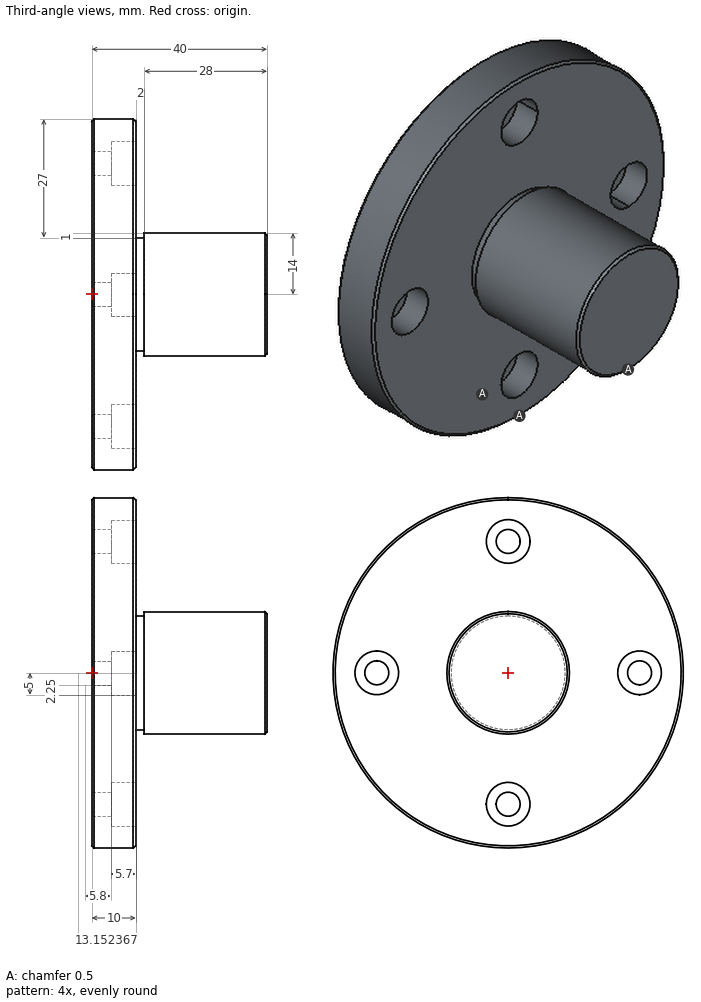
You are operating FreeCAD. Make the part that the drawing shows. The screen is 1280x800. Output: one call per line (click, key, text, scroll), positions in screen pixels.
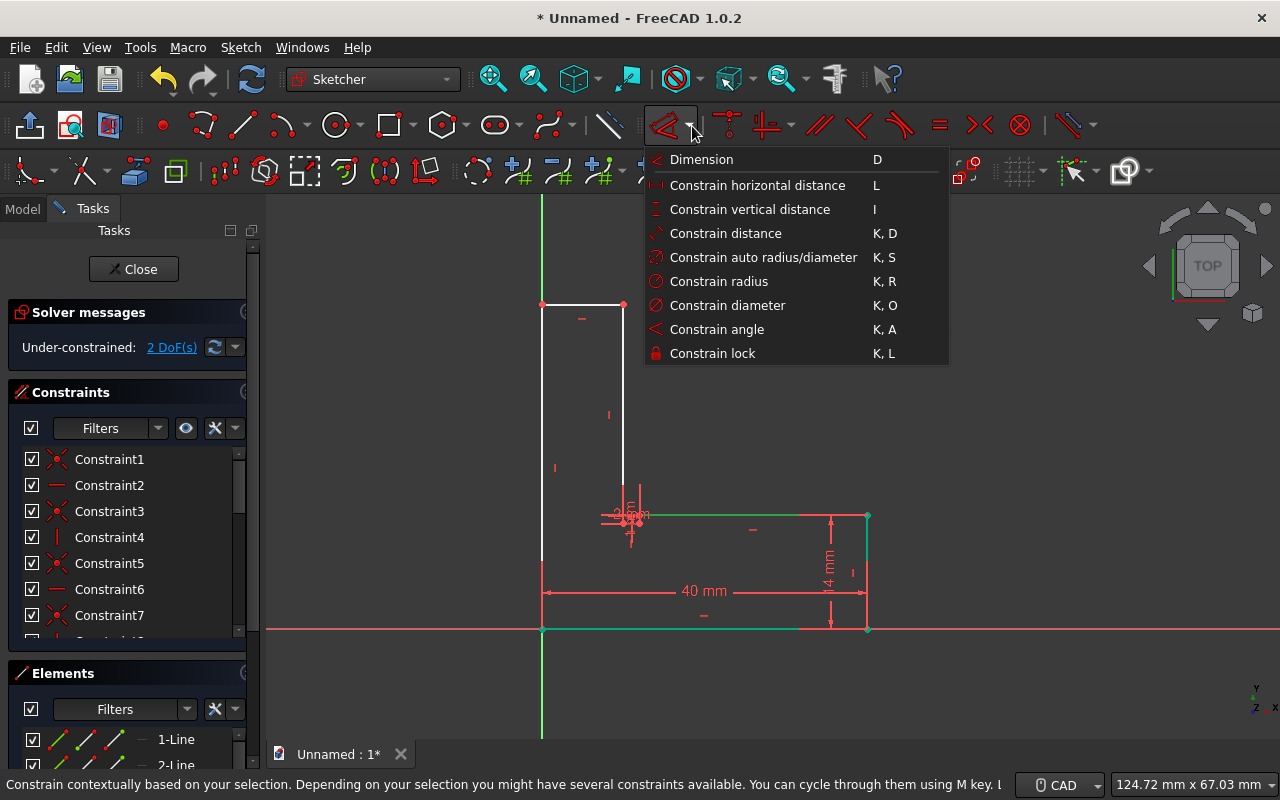
click(797, 185)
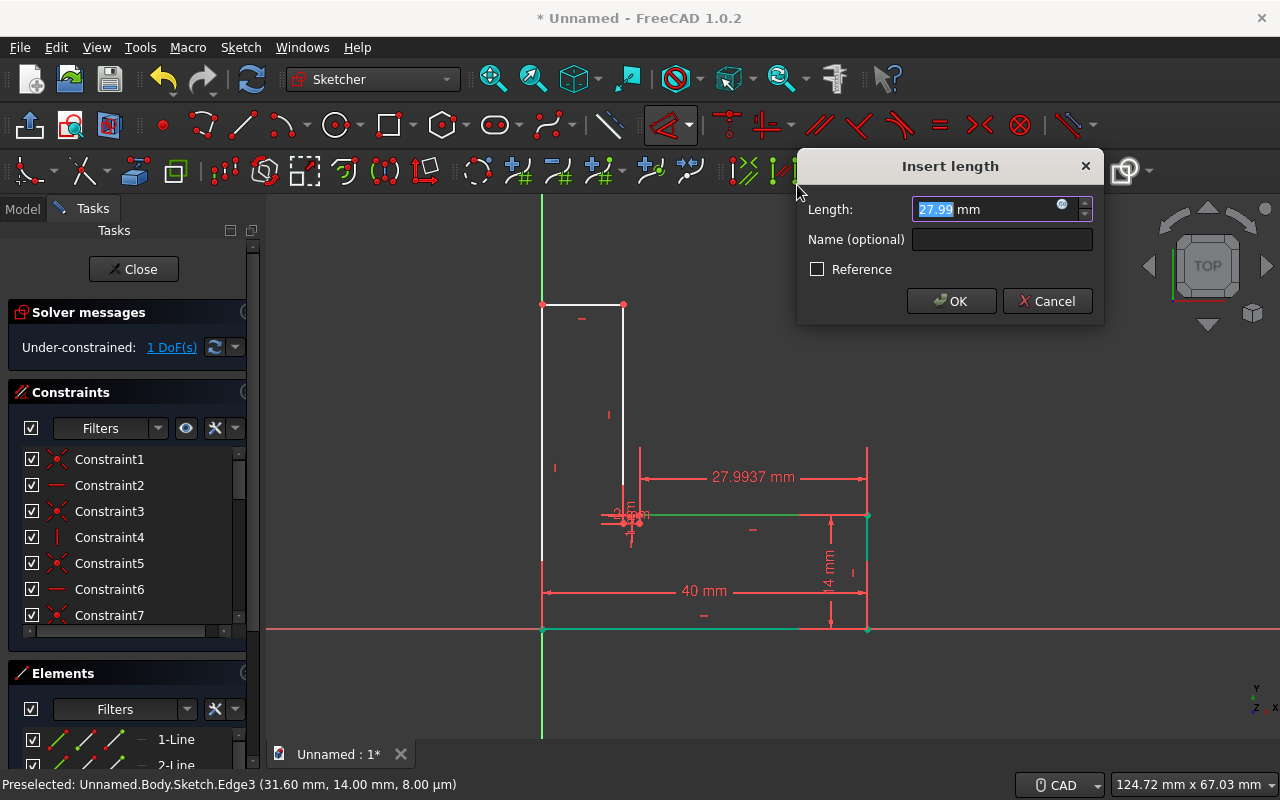
text(28)
key(Return)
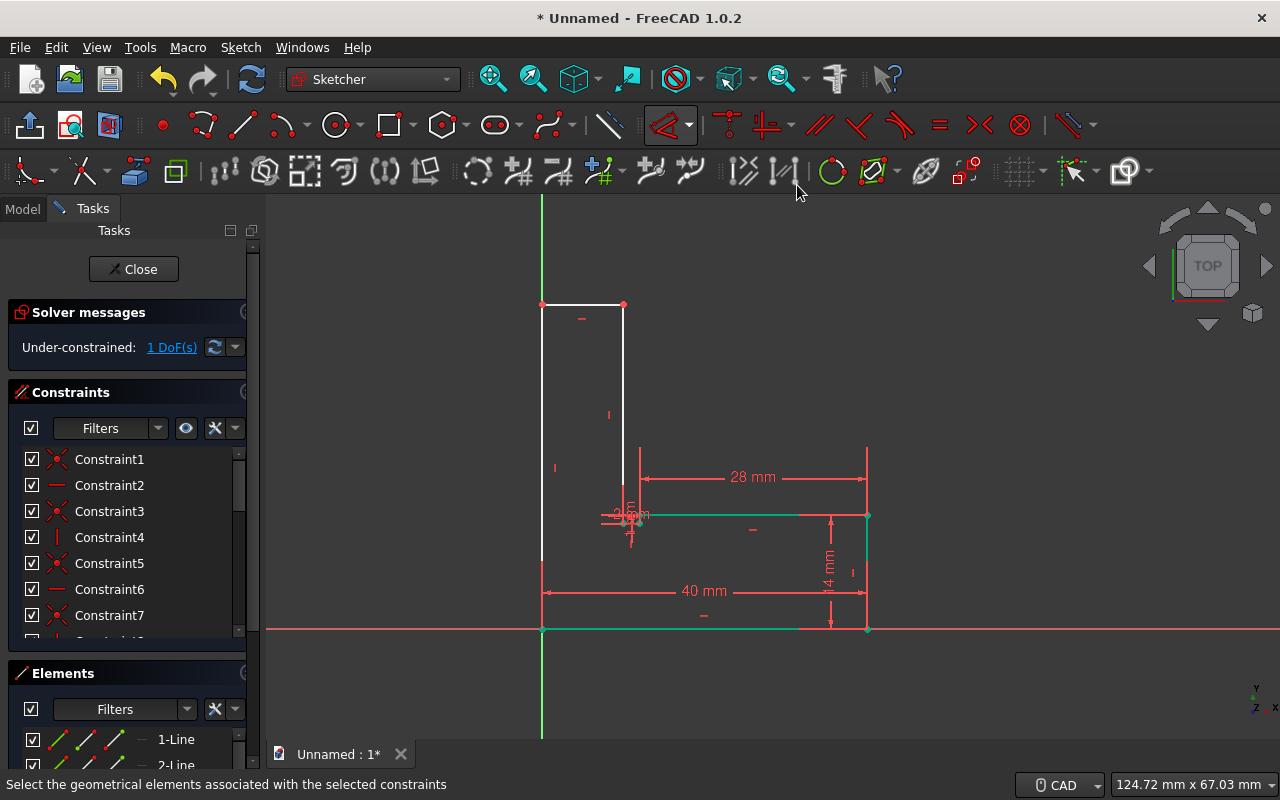
click(623, 458)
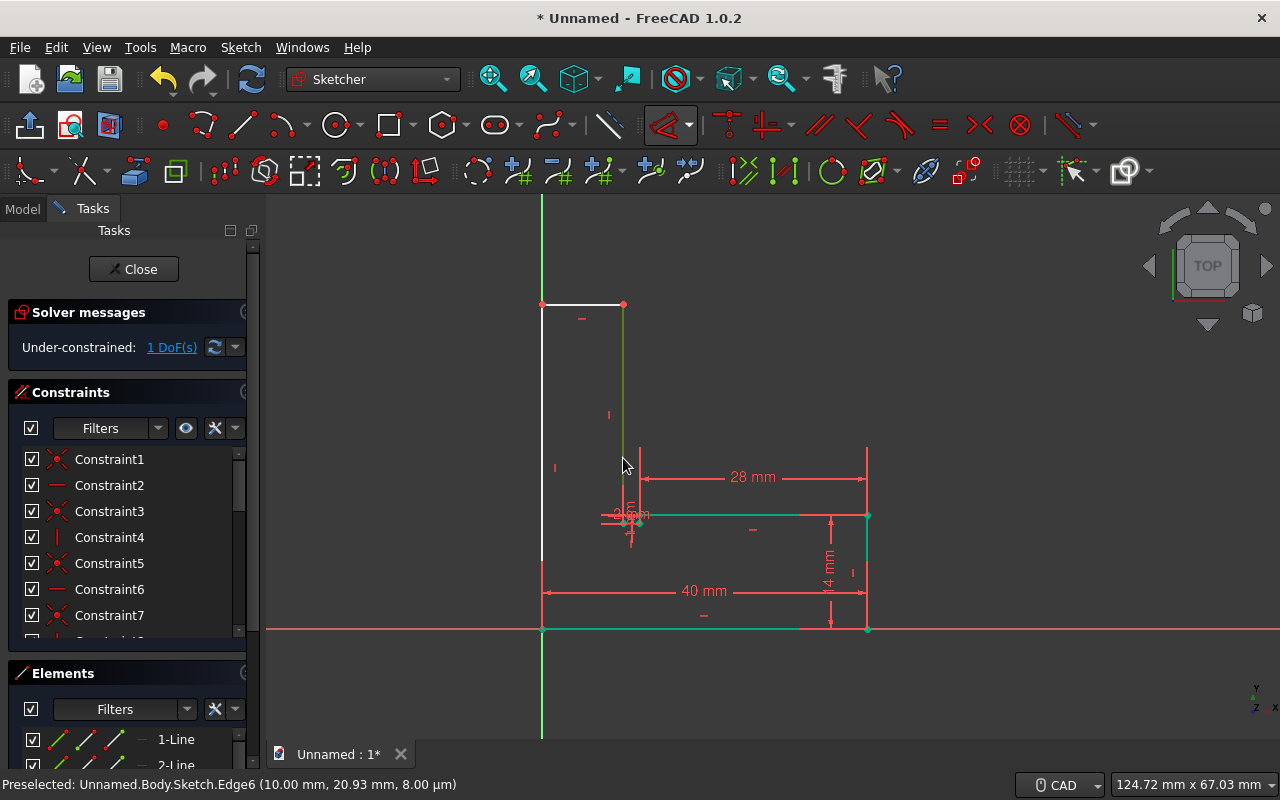
click(692, 126)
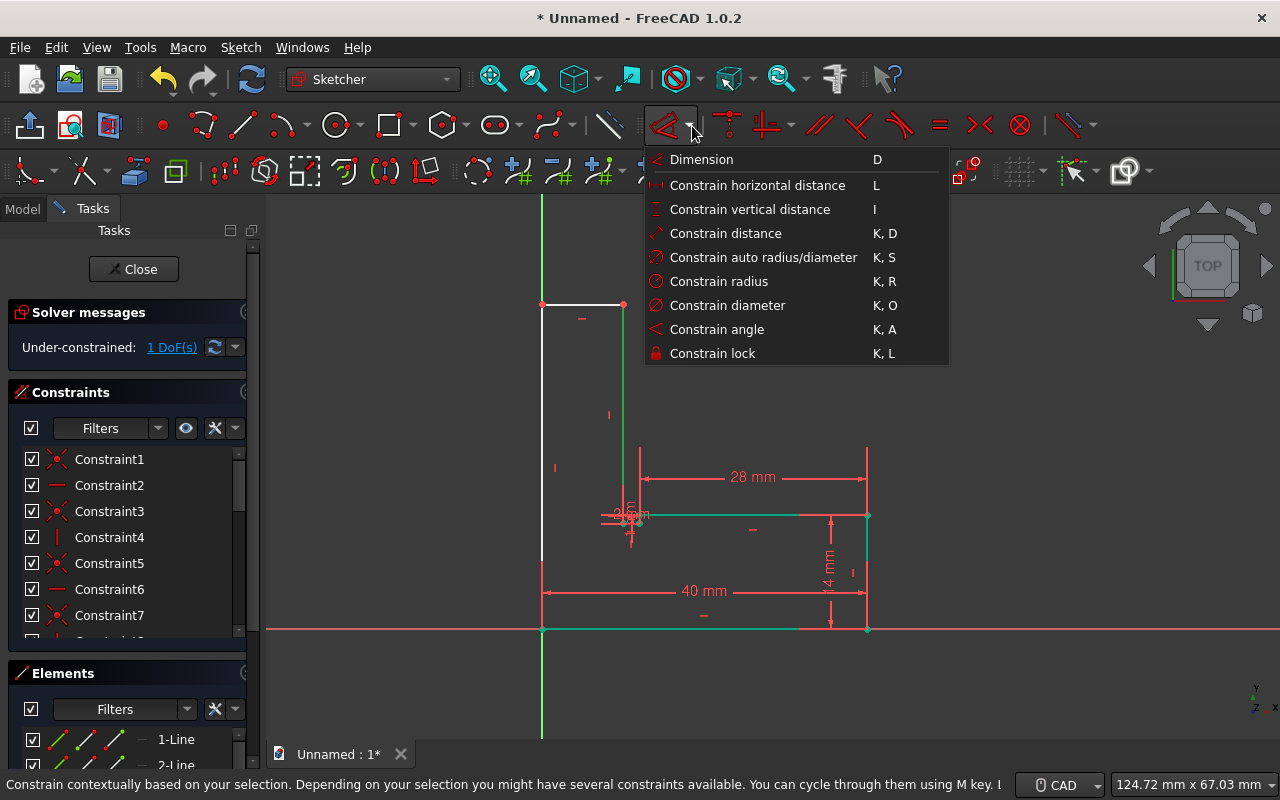
click(797, 209)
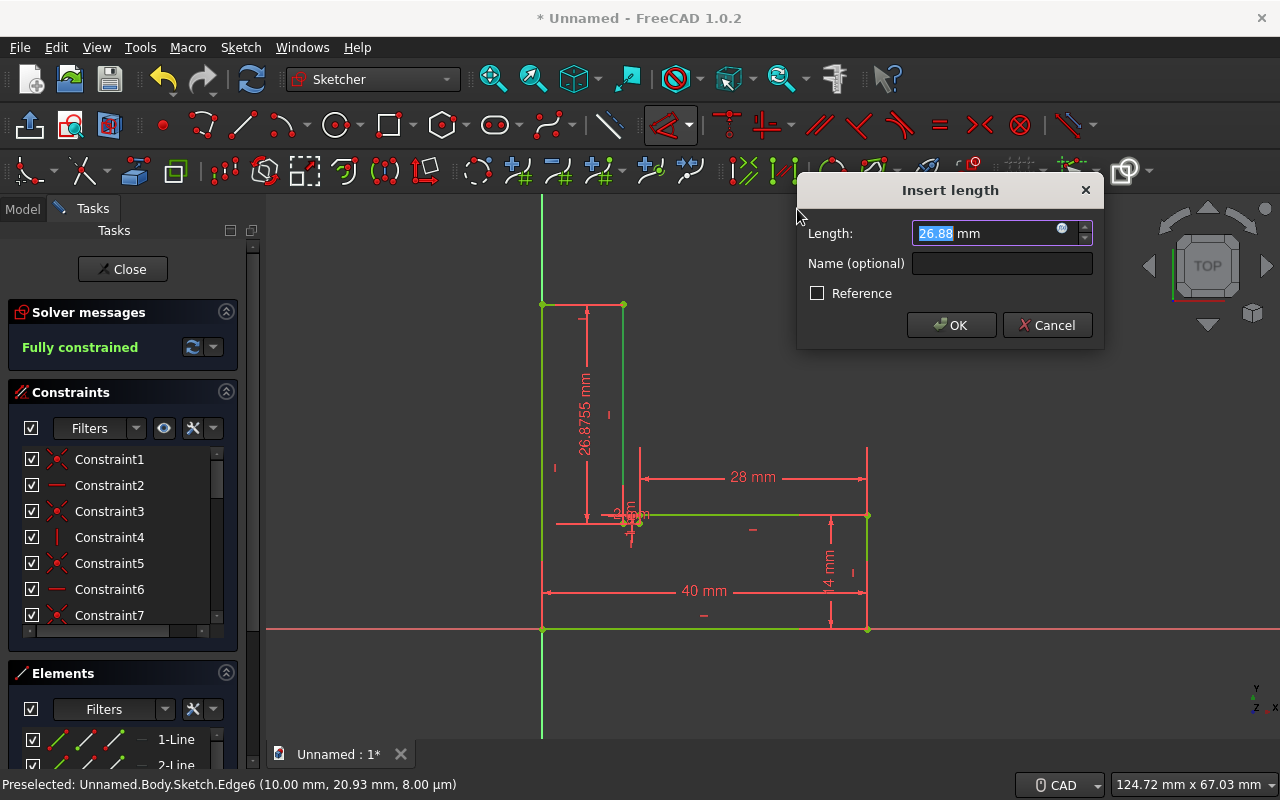
text(27)
key(Return)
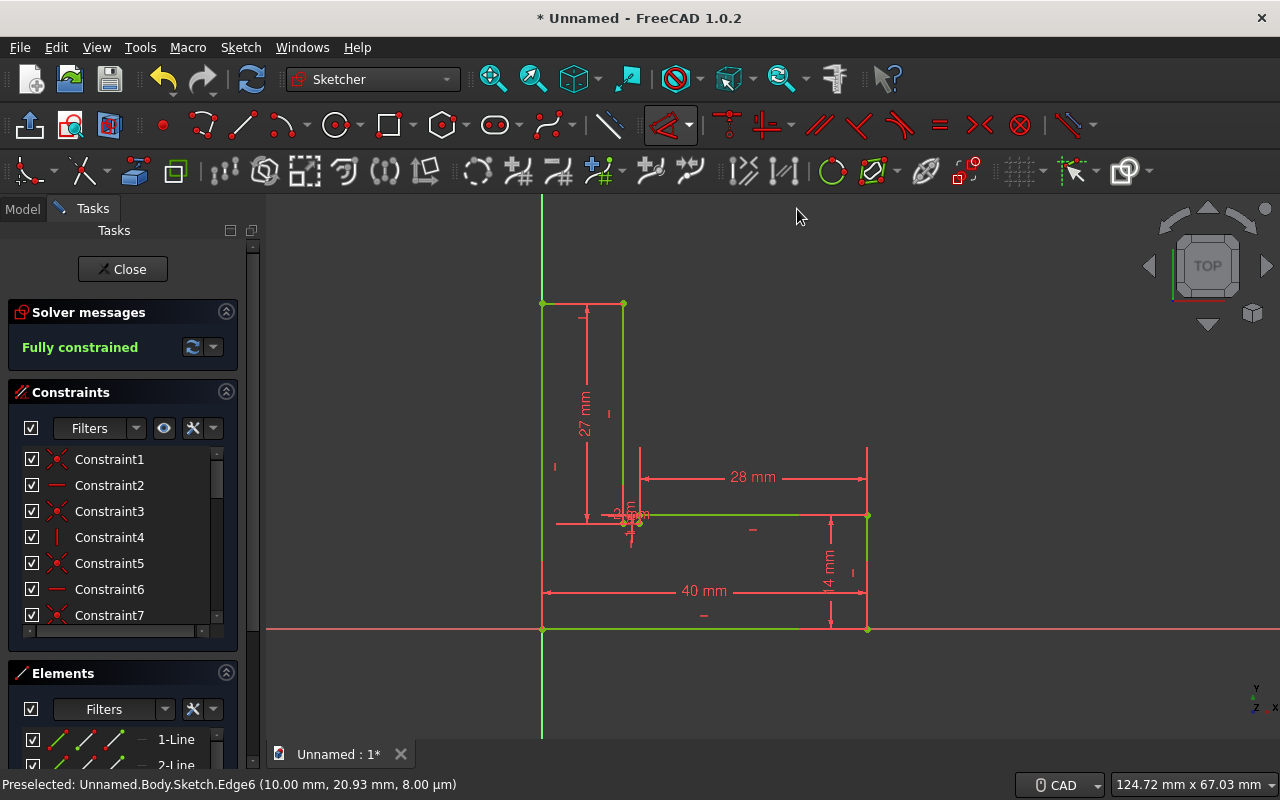
click(123, 269)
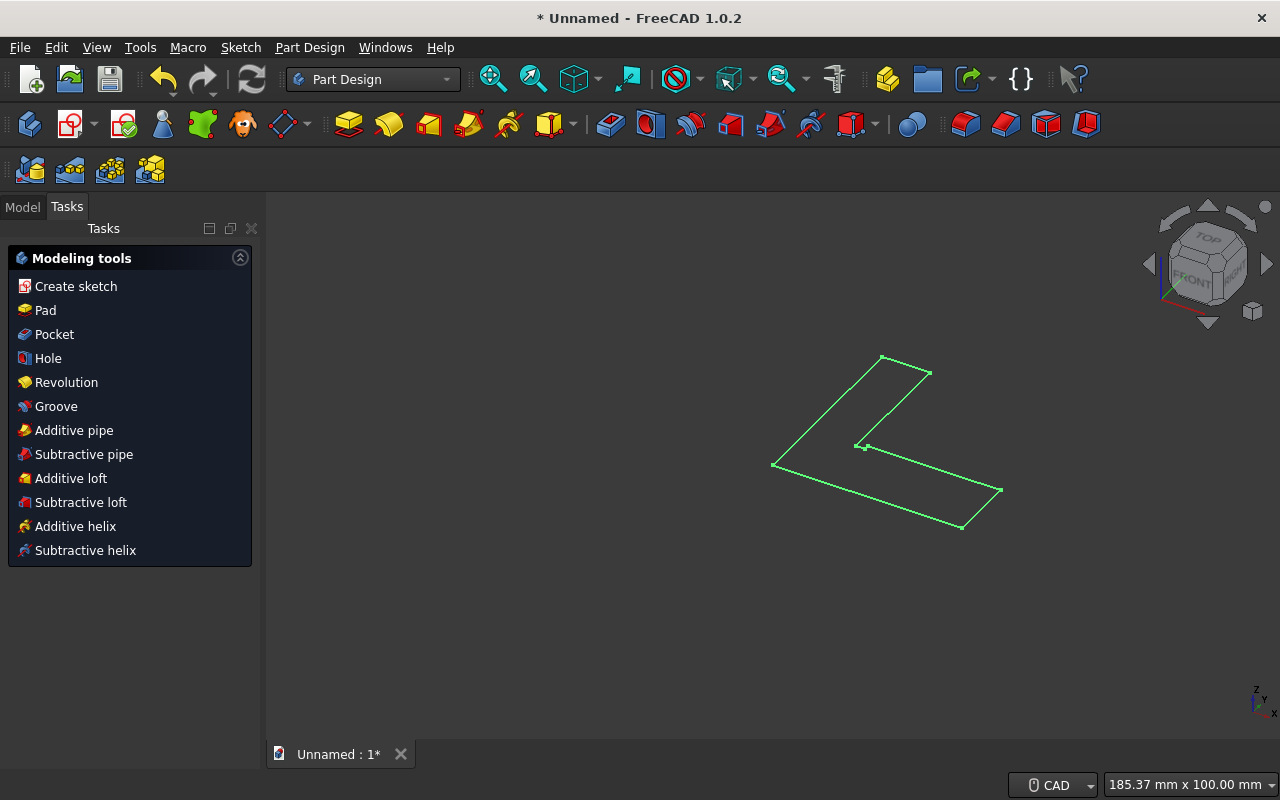
click(390, 124)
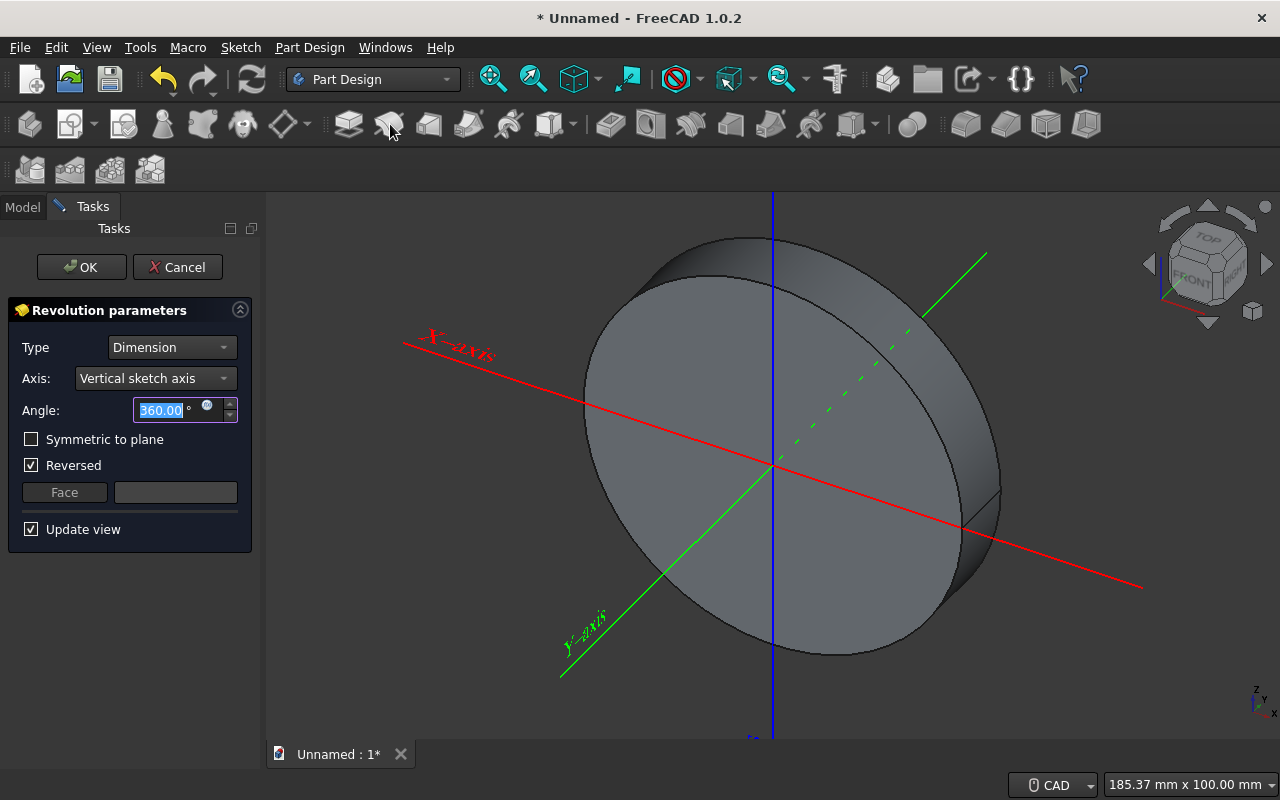
click(156, 378)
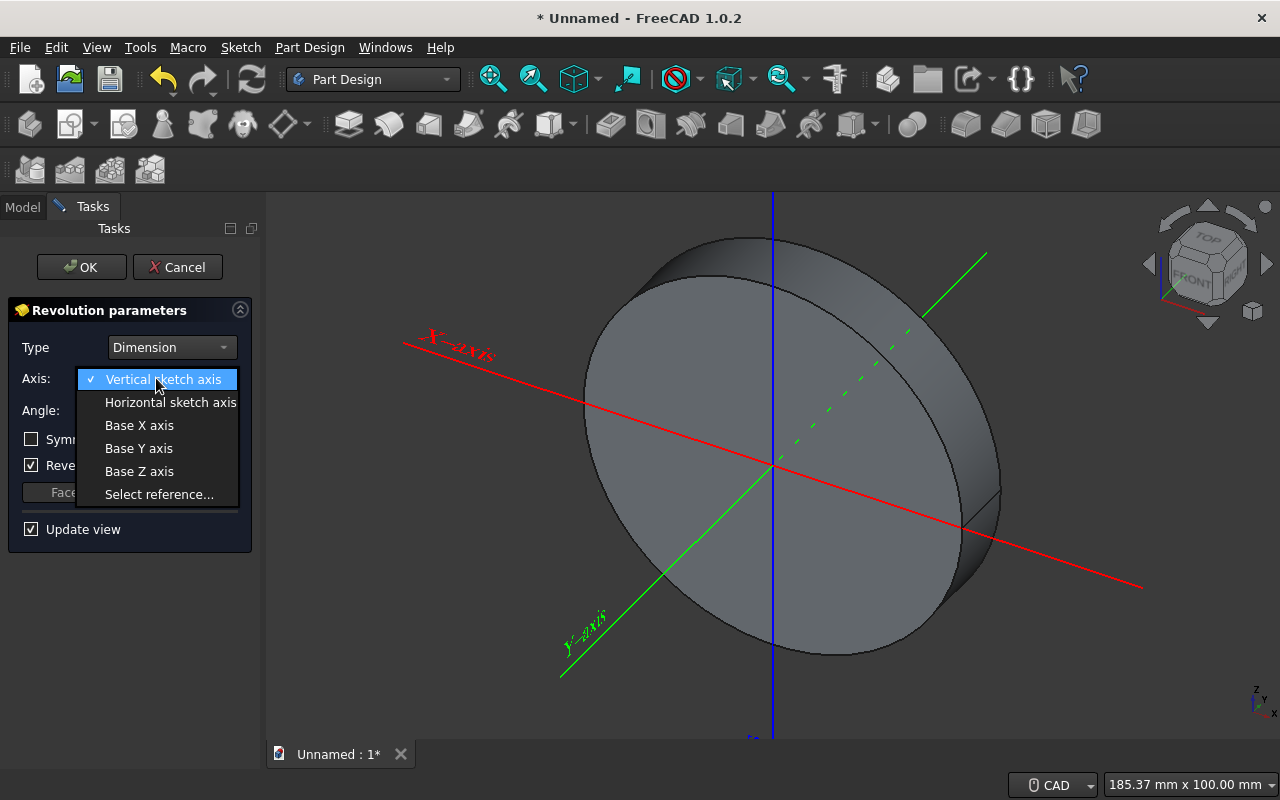
click(156, 402)